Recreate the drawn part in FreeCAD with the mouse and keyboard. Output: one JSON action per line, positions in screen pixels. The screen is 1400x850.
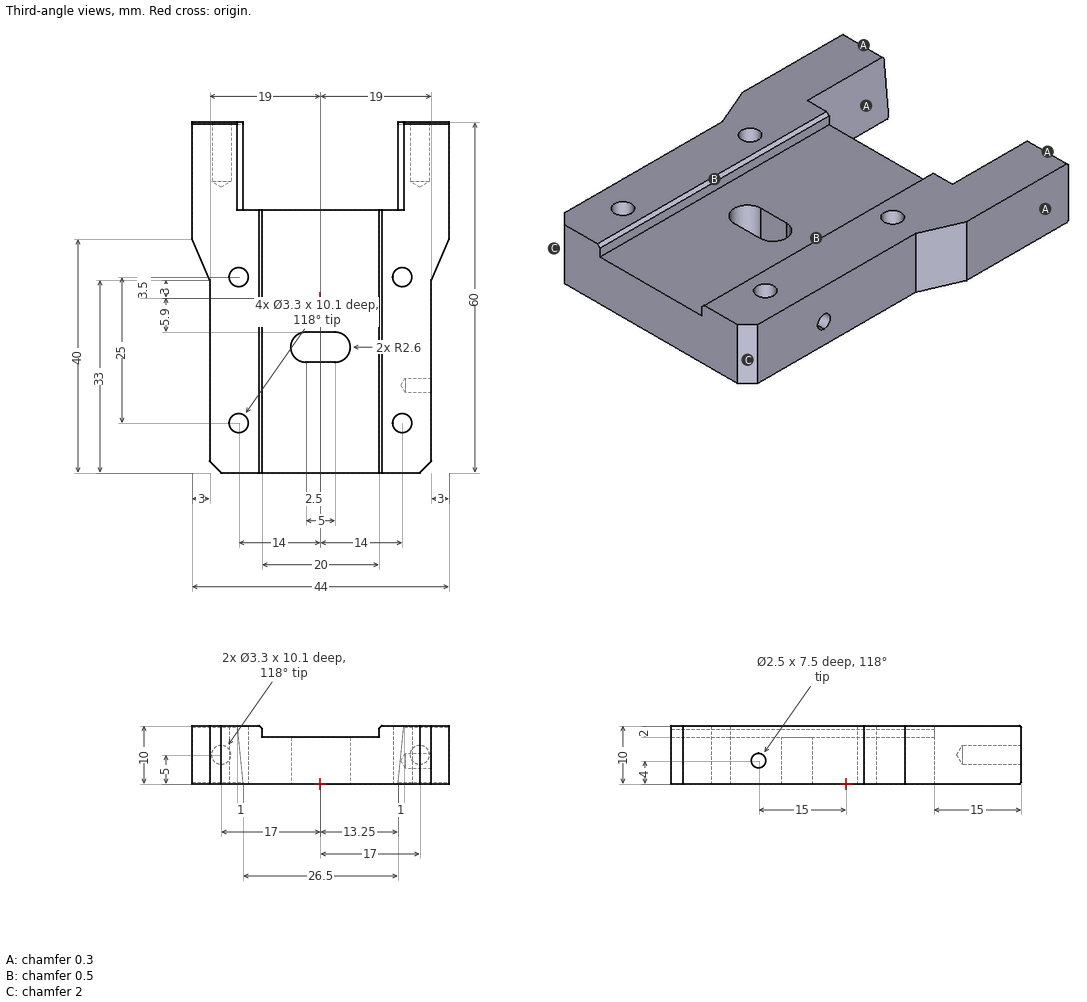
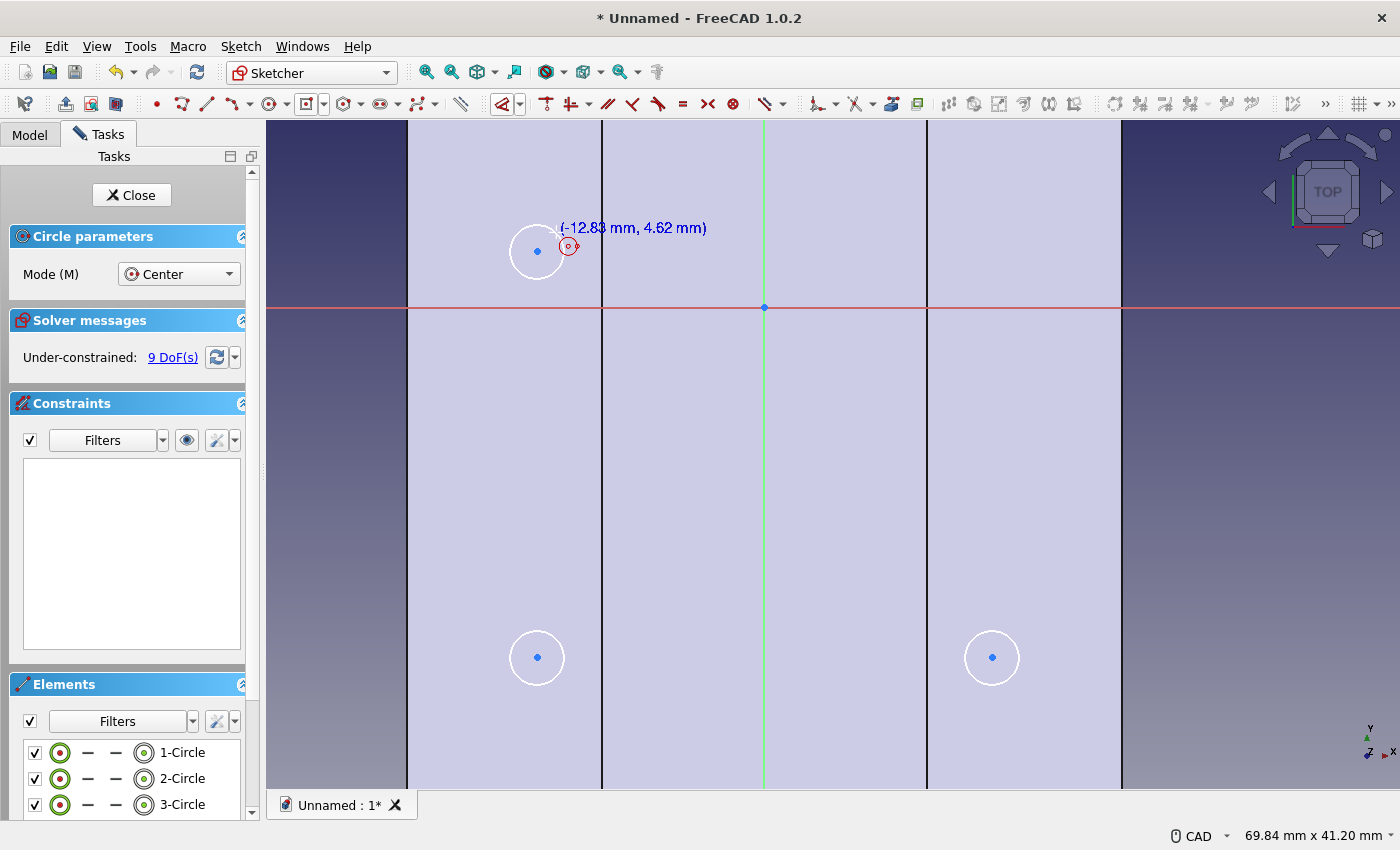
{"action": "left_click", "coordinate": [992, 251]}
{"action": "left_click", "coordinate": [1011, 232]}
{"action": "key", "text": "Escape"}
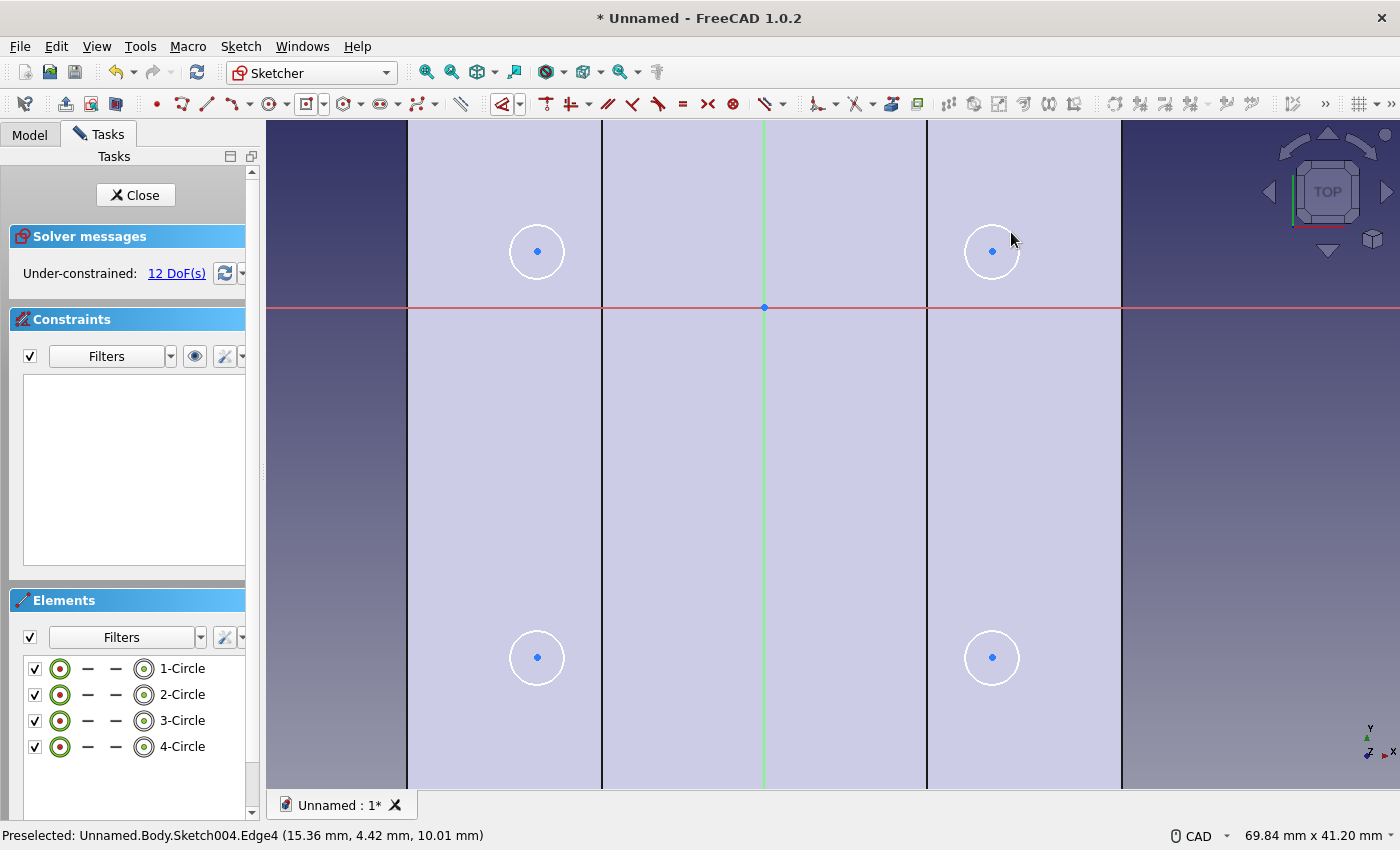
{"action": "left_click", "coordinate": [556, 639]}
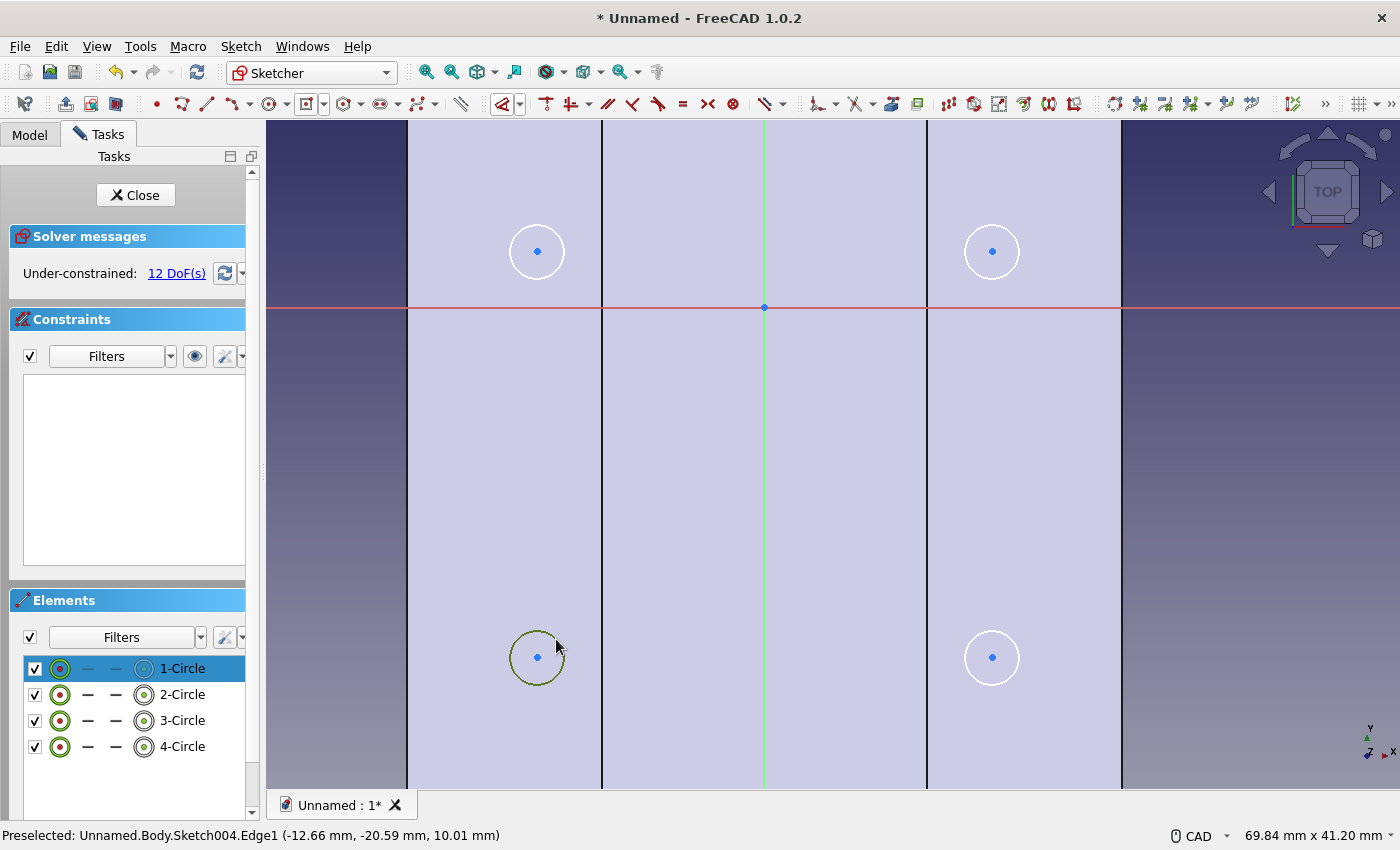
{"action": "left_click", "coordinate": [1011, 639]}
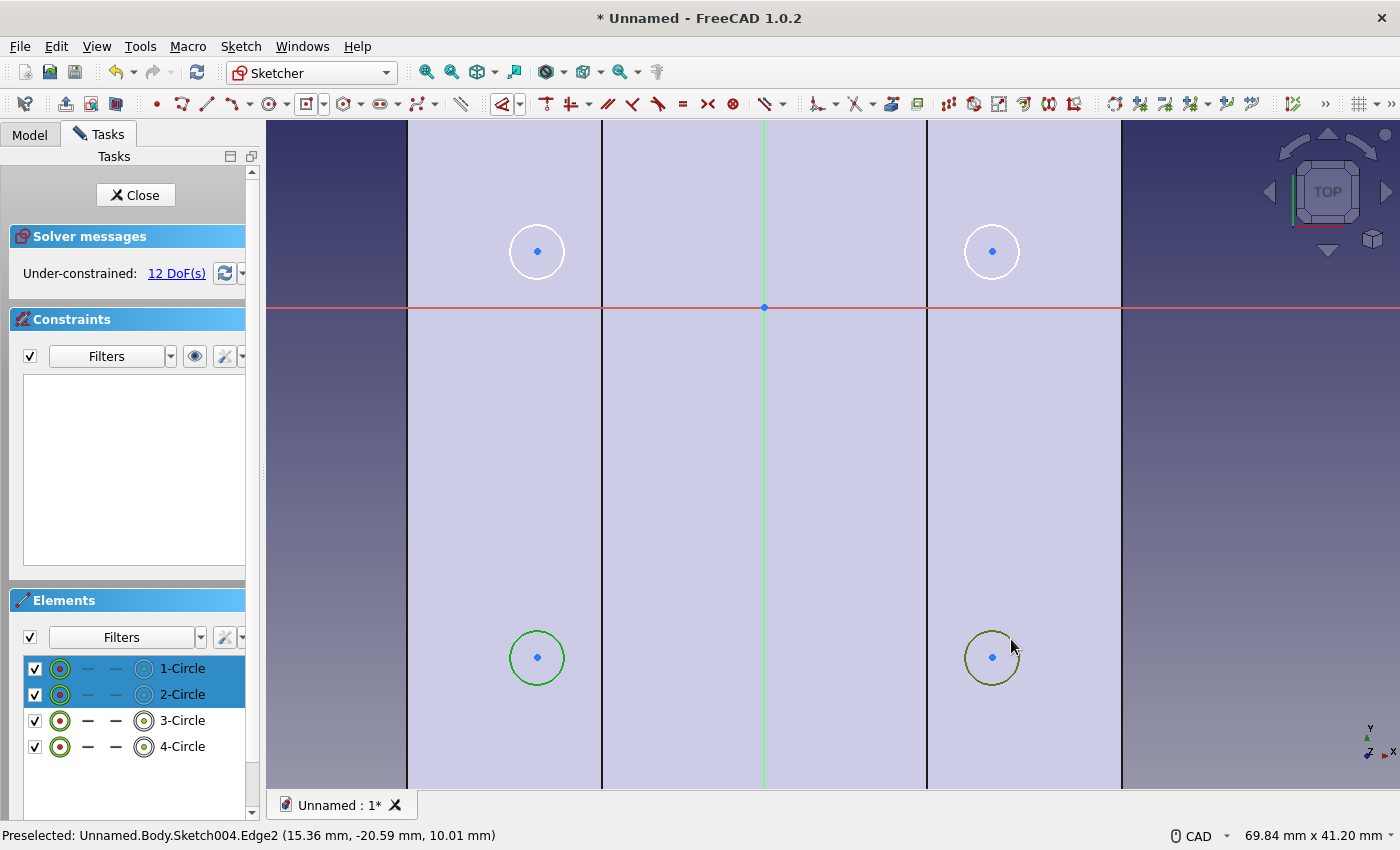
{"action": "left_click", "coordinate": [556, 233]}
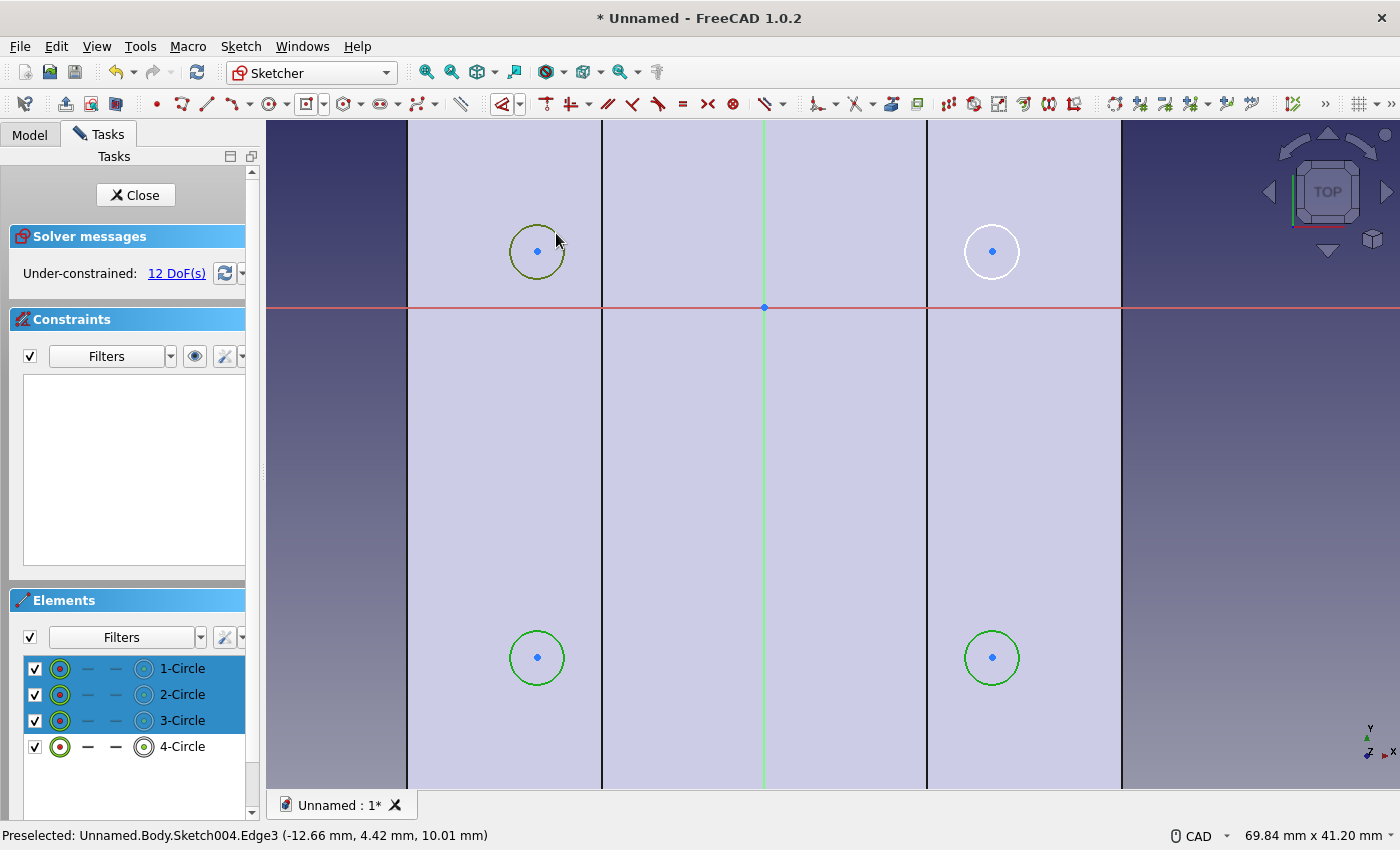
{"action": "left_click", "coordinate": [1011, 233]}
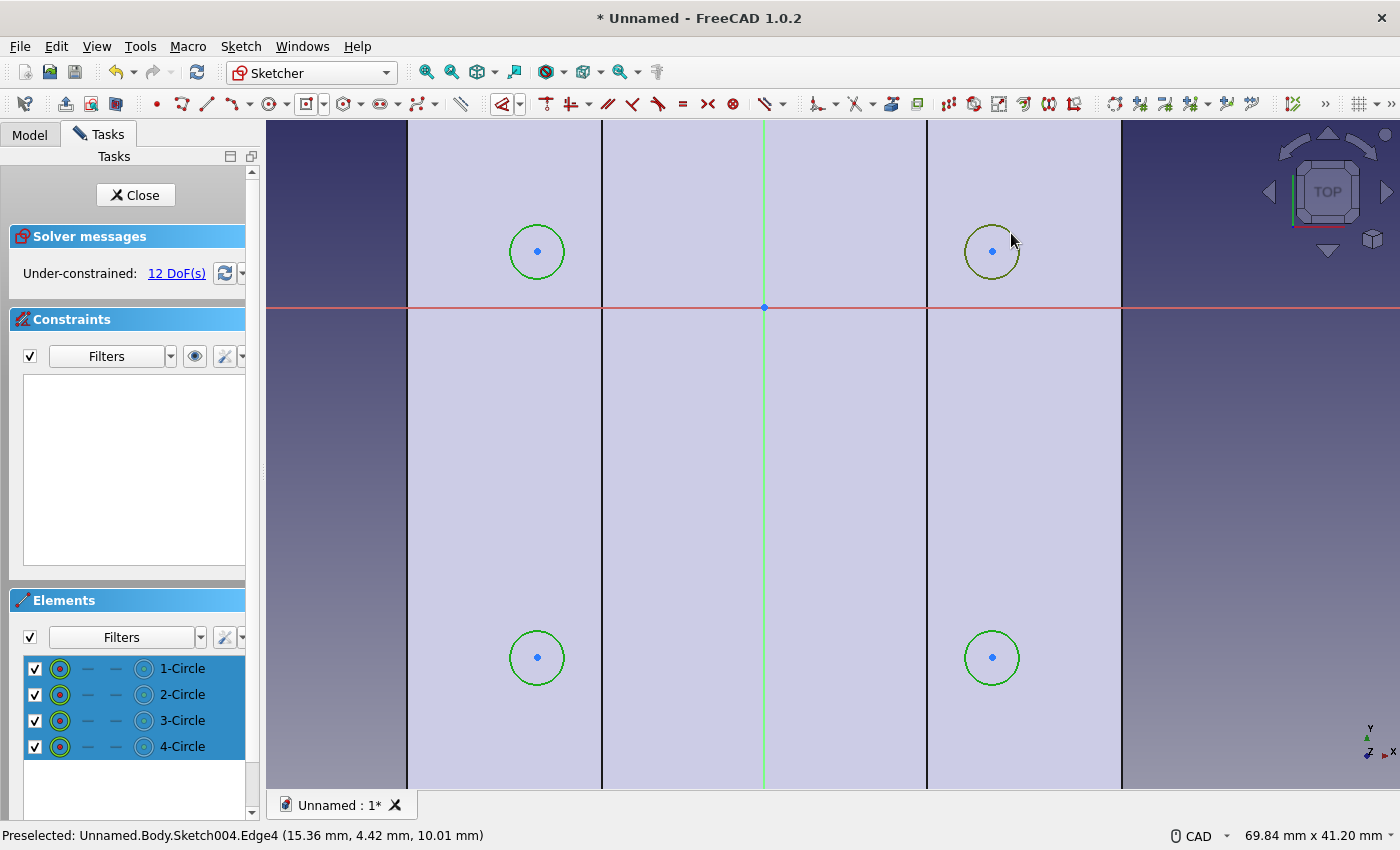
{"action": "left_click", "coordinate": [683, 104]}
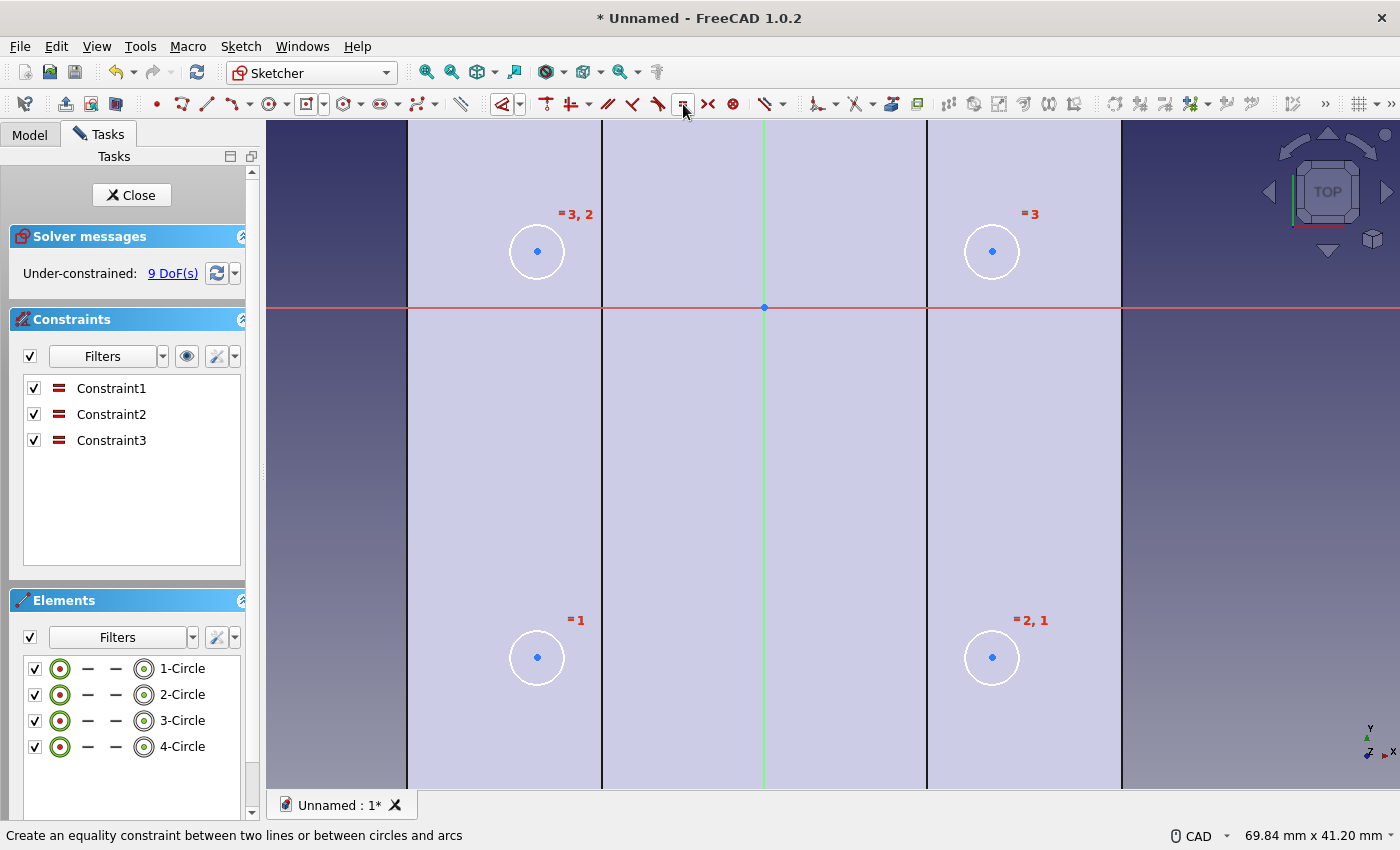
{"action": "left_click", "coordinate": [556, 639]}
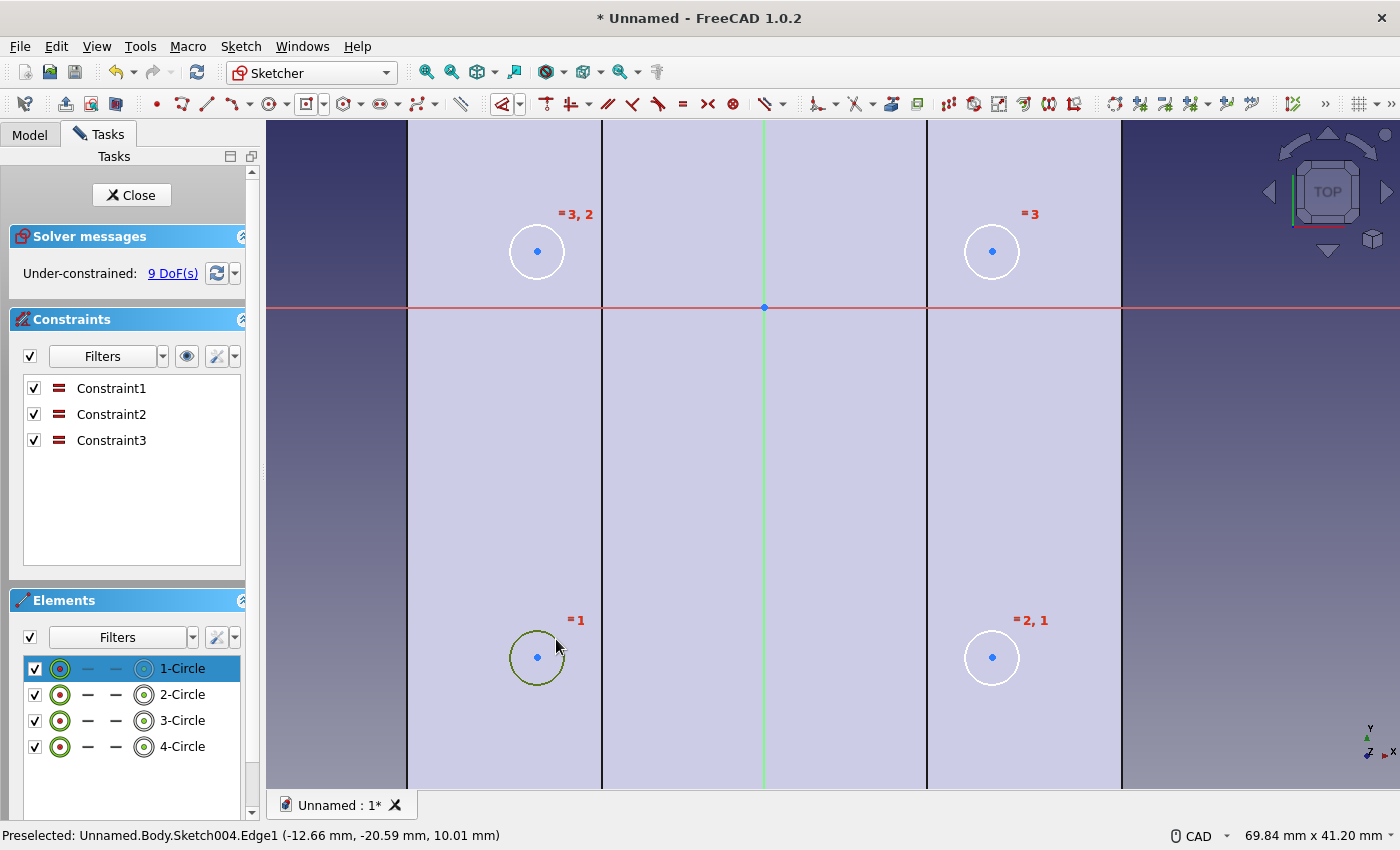
{"action": "key", "text": "k o"}